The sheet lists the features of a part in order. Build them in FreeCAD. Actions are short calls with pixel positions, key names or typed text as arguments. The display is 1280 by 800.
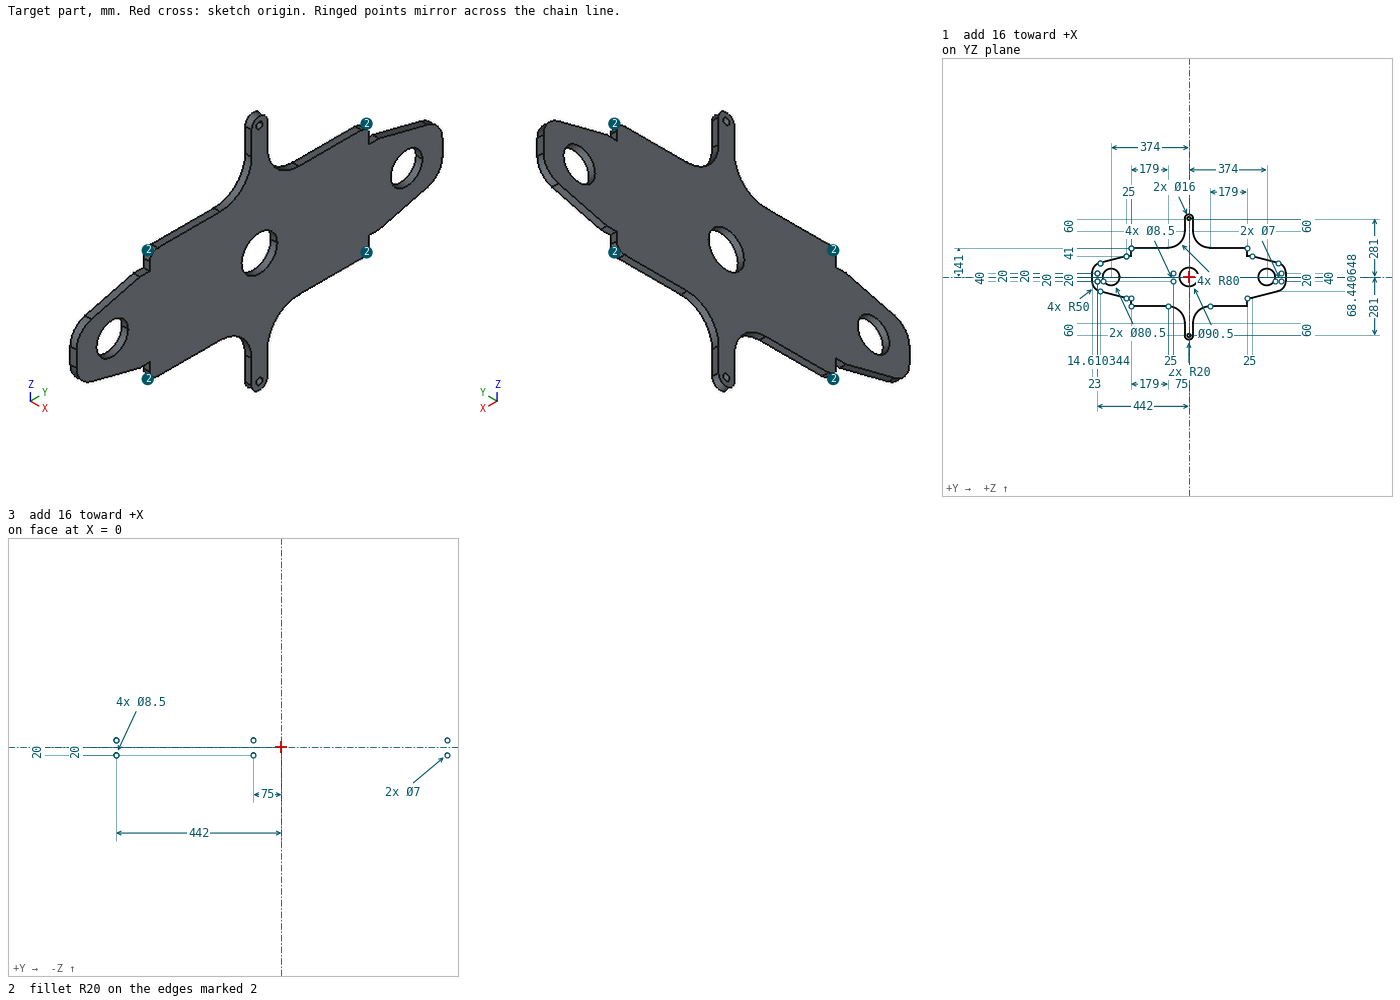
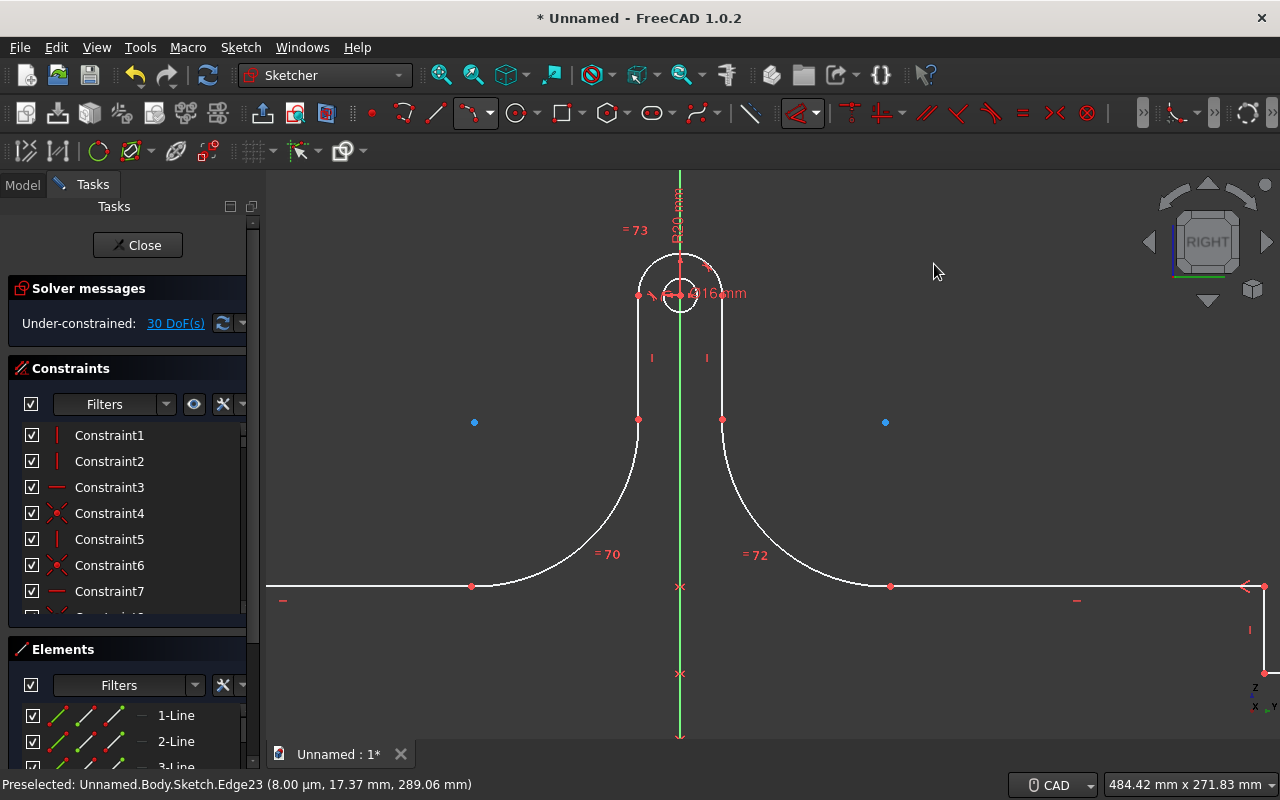
click(548, 569)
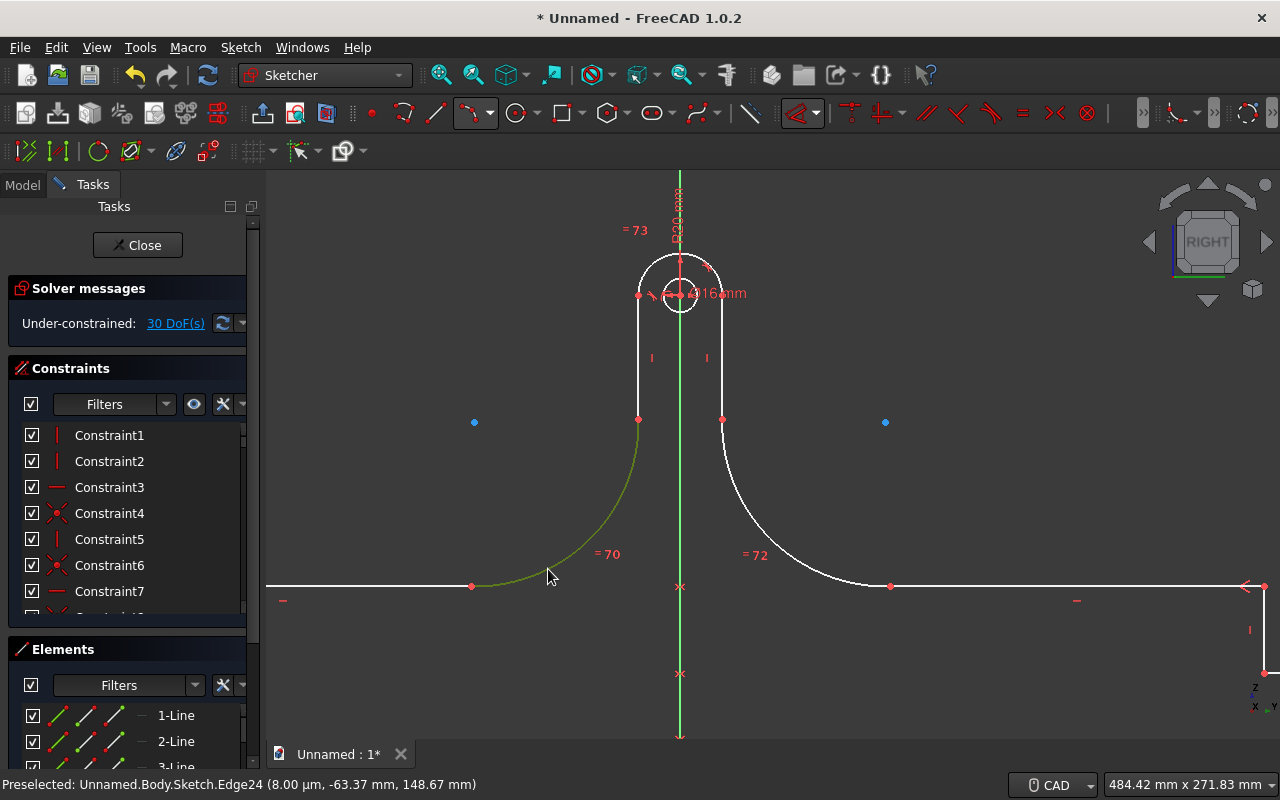
key(k)
key(r)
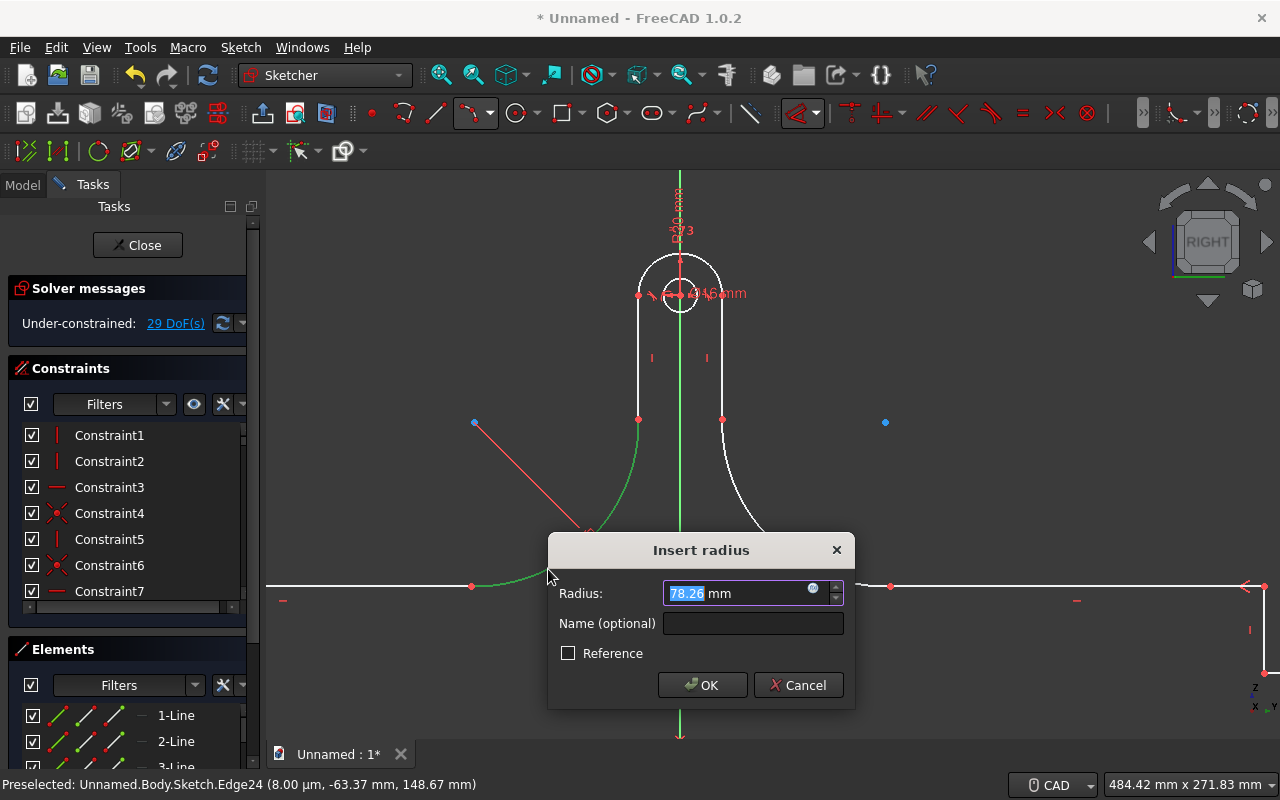
text(80)
key(Return)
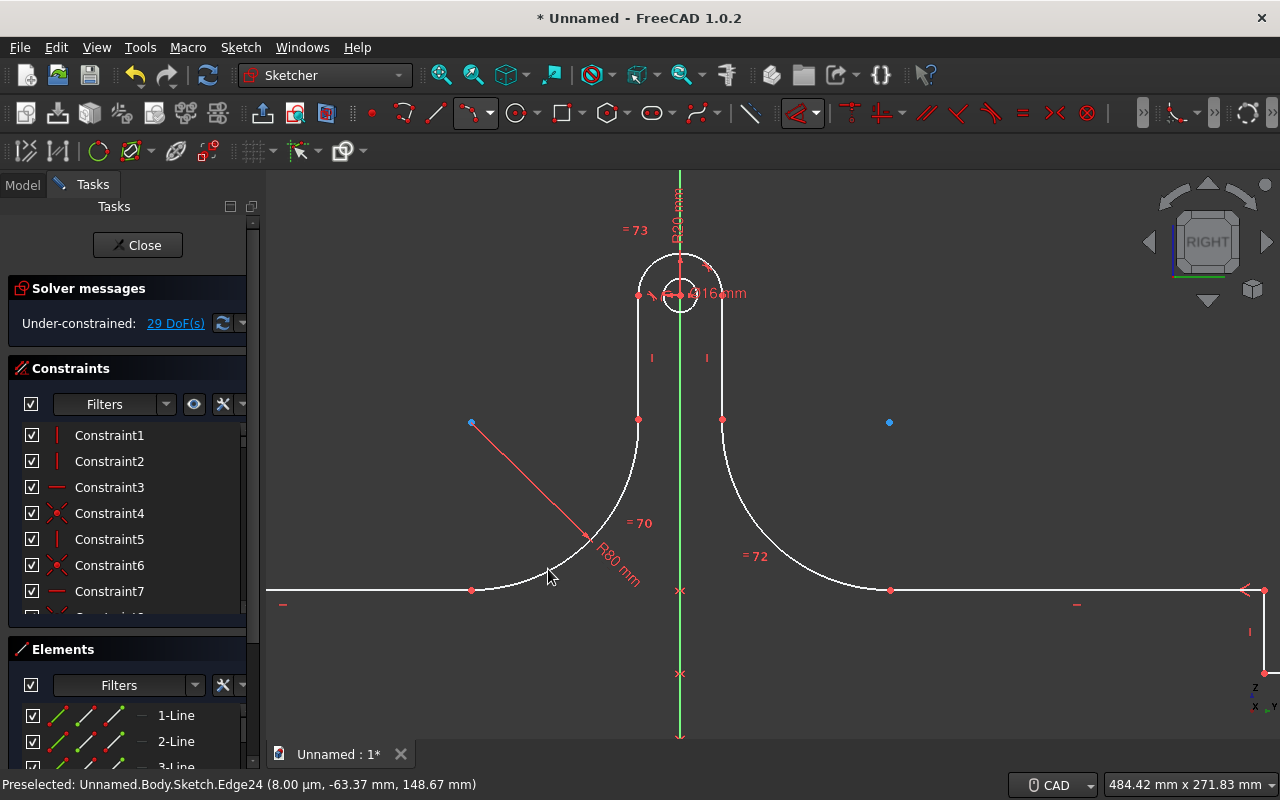
scroll(715, 271, down, 6)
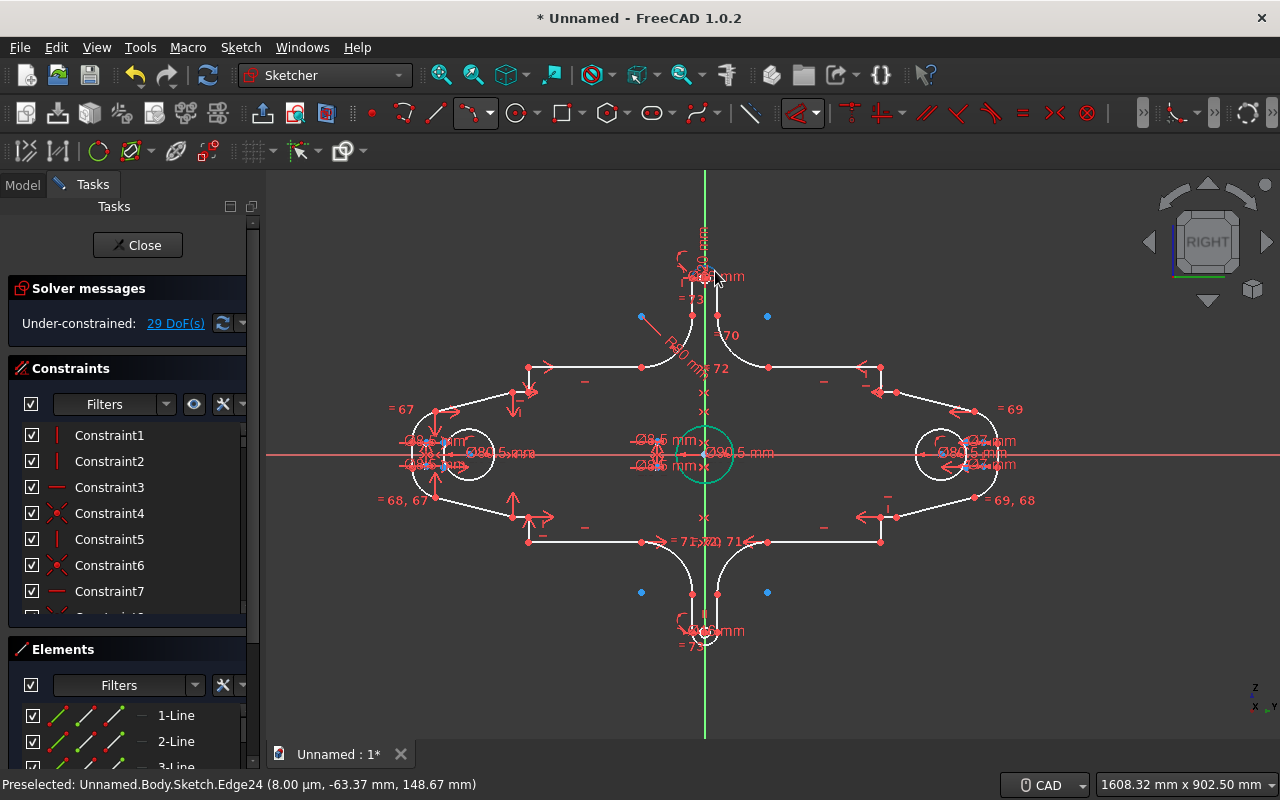
scroll(424, 417, up, 2)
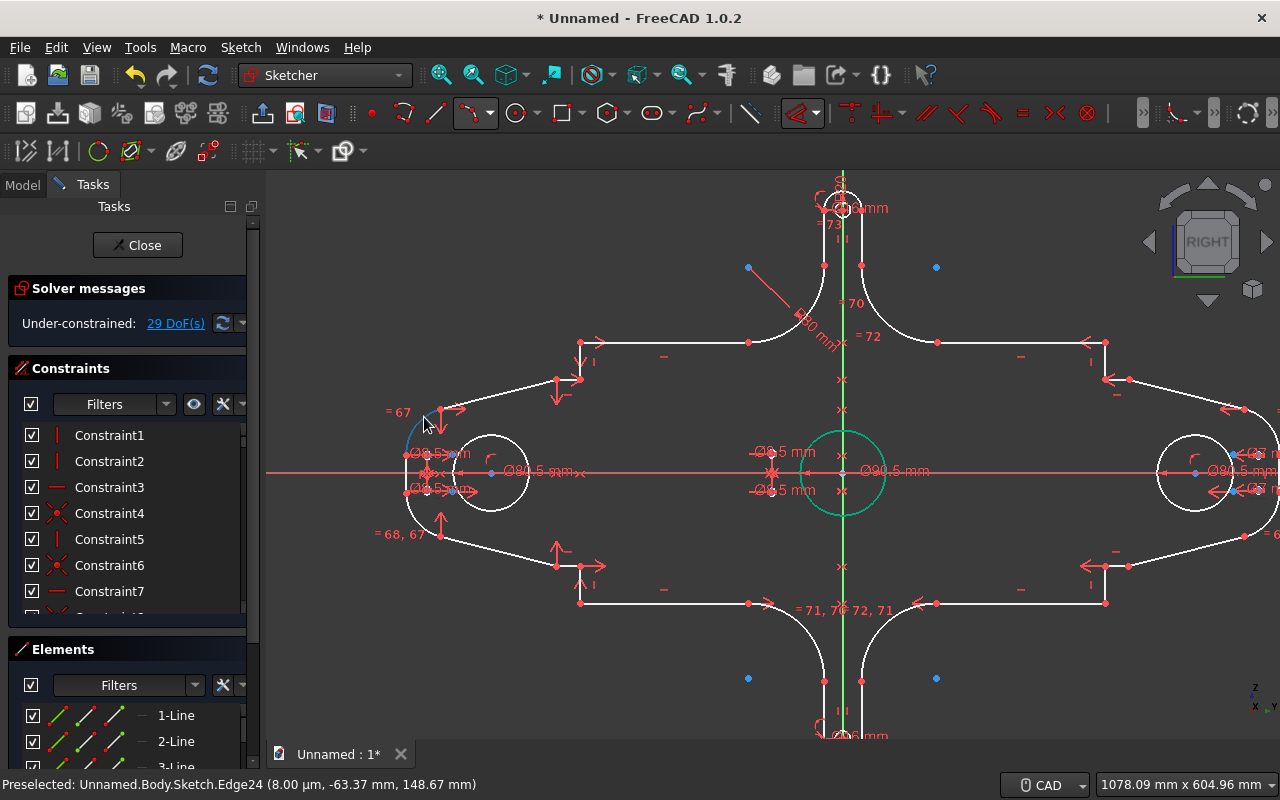
click(424, 417)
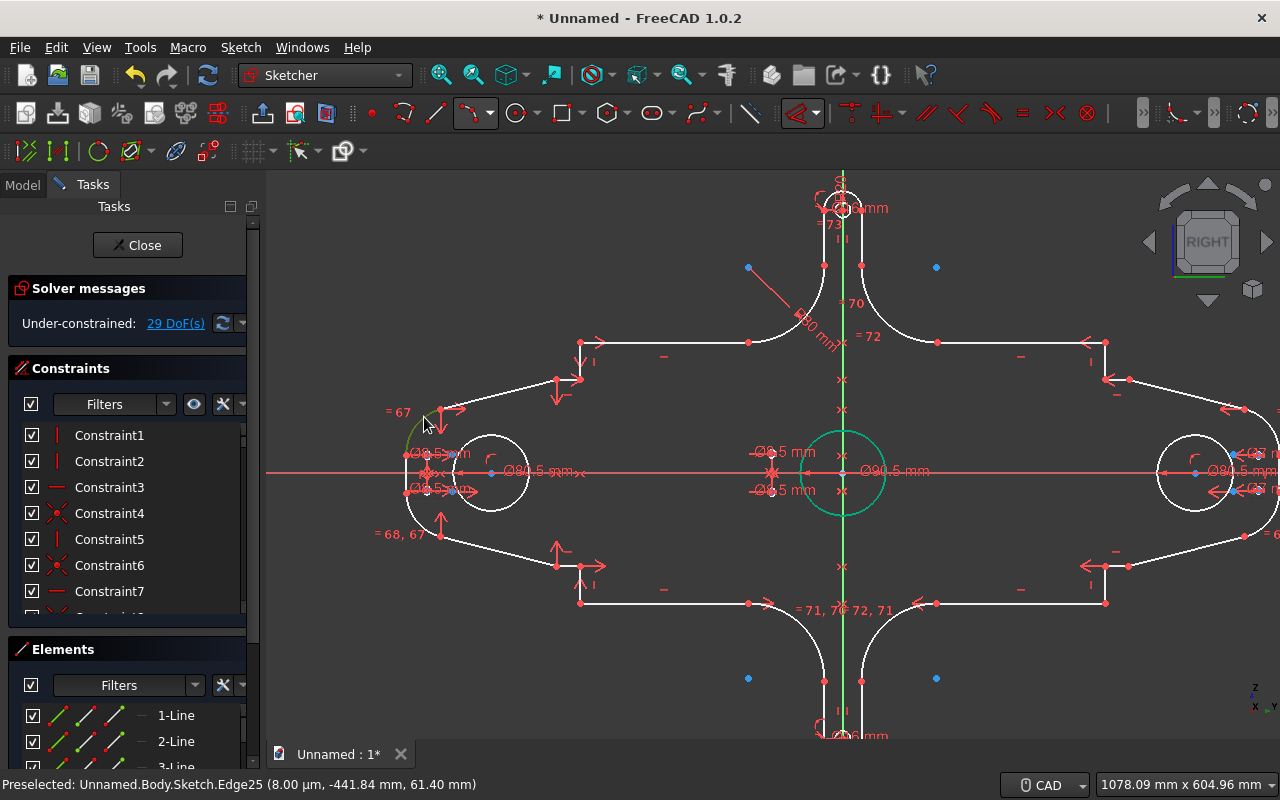
click(818, 114)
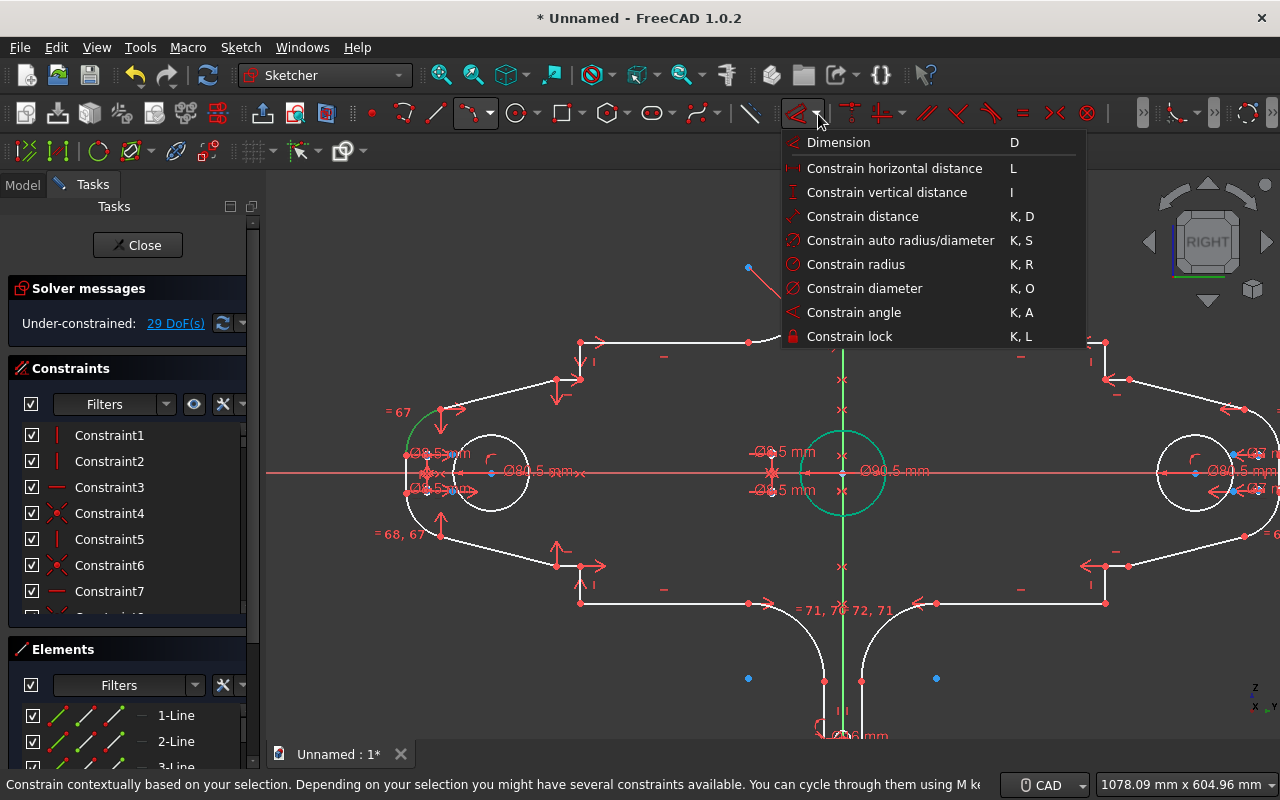
click(934, 264)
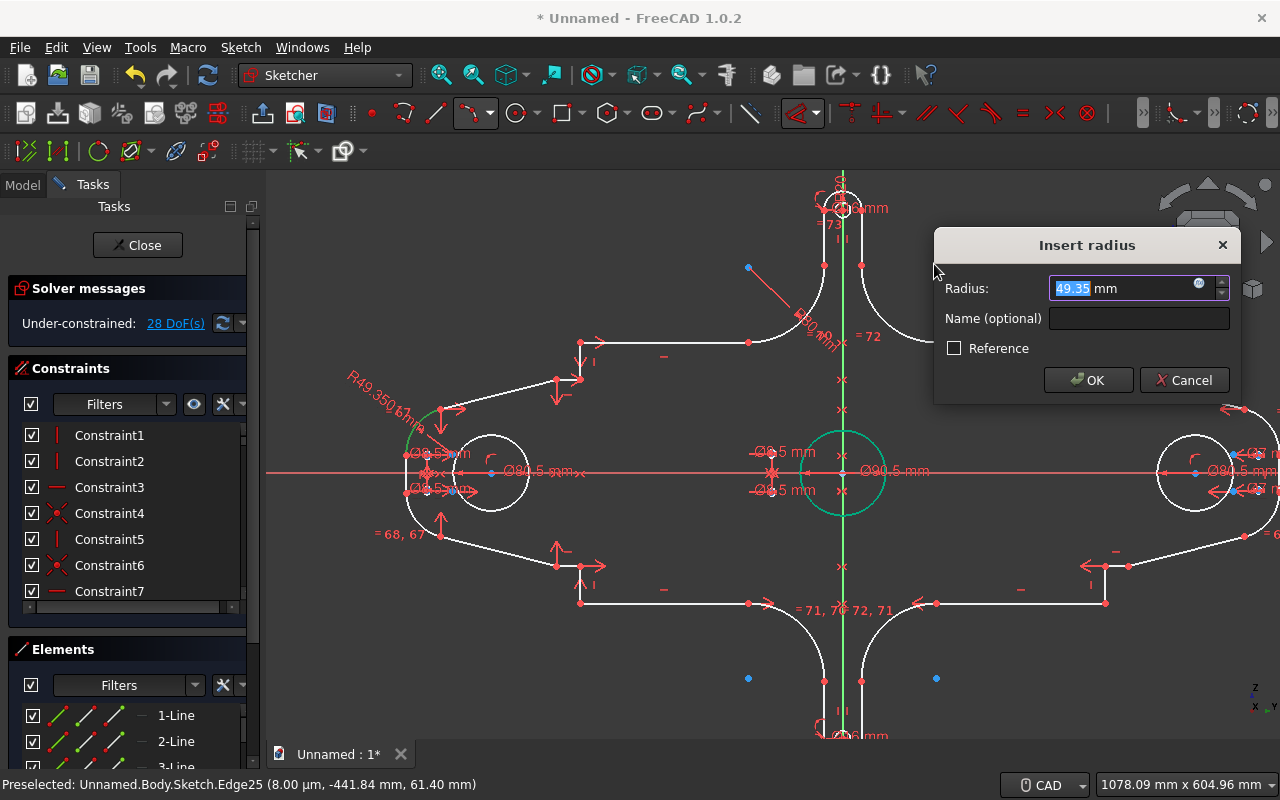
text(50)
key(Return)